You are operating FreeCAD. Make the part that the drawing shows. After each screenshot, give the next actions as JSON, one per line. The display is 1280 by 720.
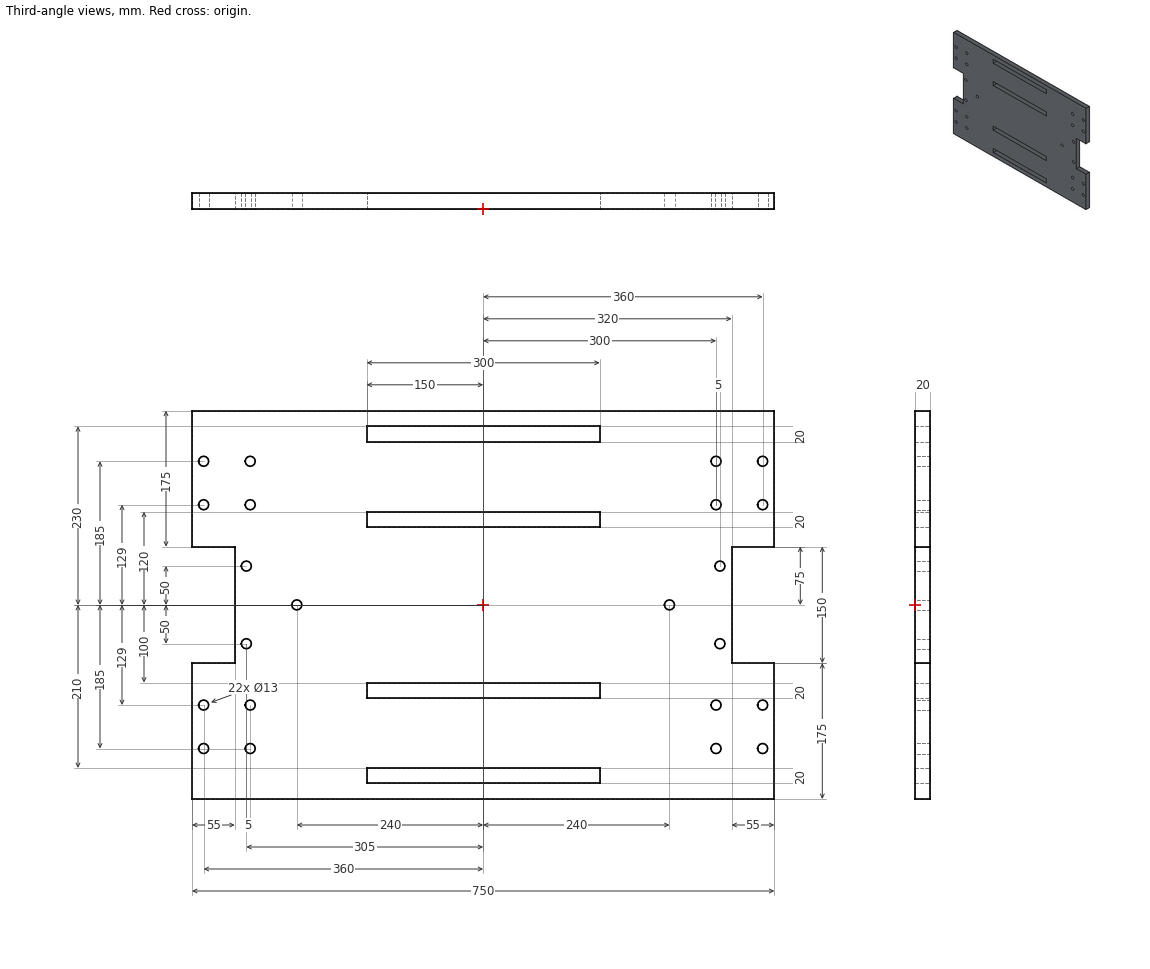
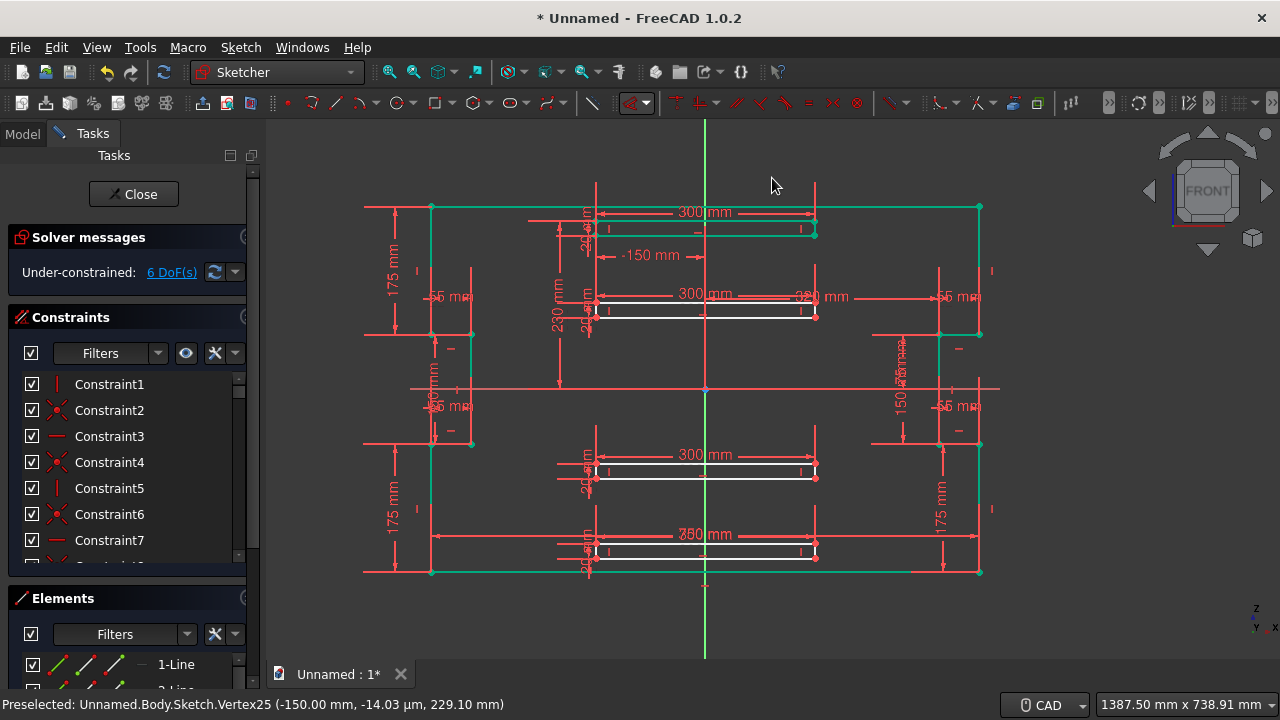
{"action": "left_click", "coordinate": [596, 303]}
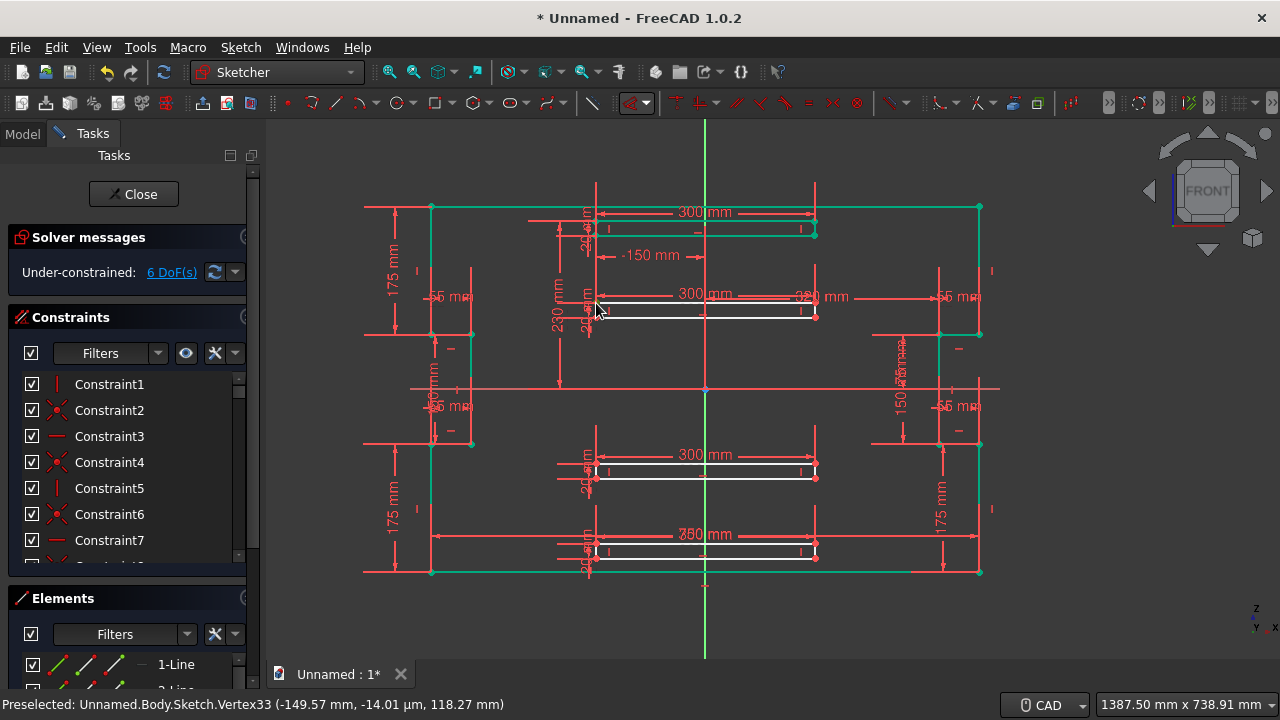
{"action": "left_click", "coordinate": [648, 104]}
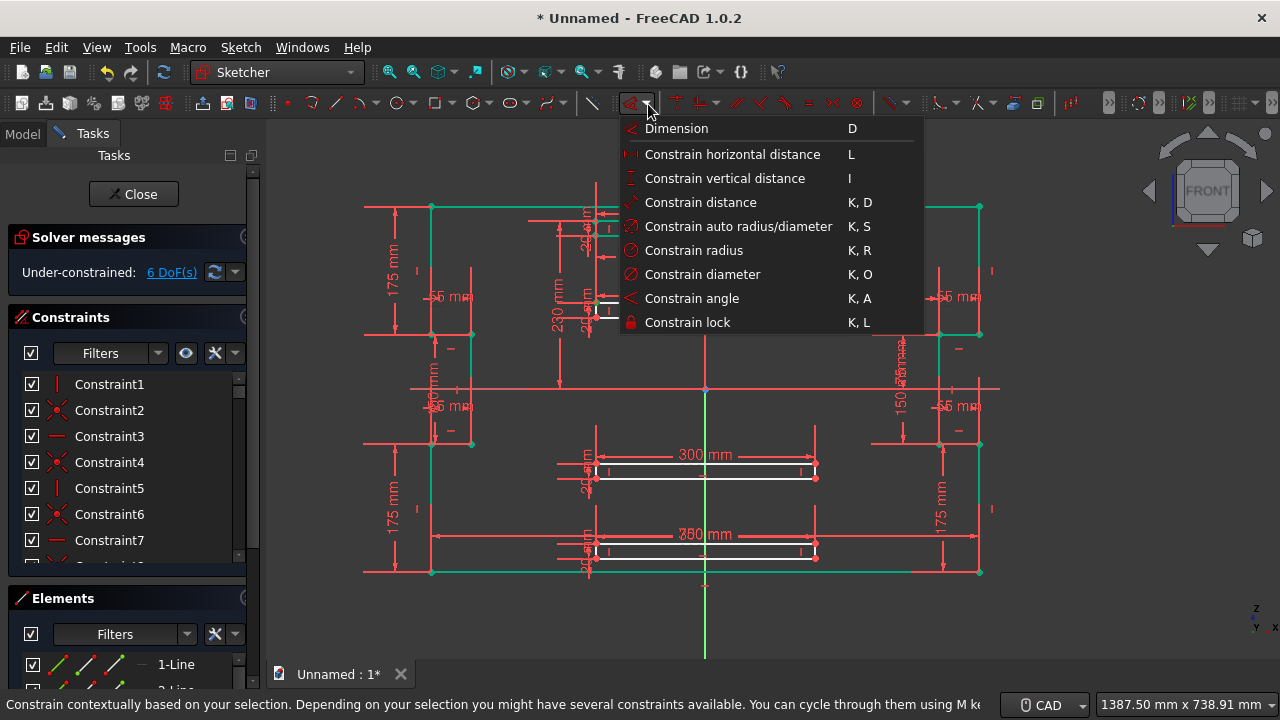
{"action": "left_click", "coordinate": [772, 154]}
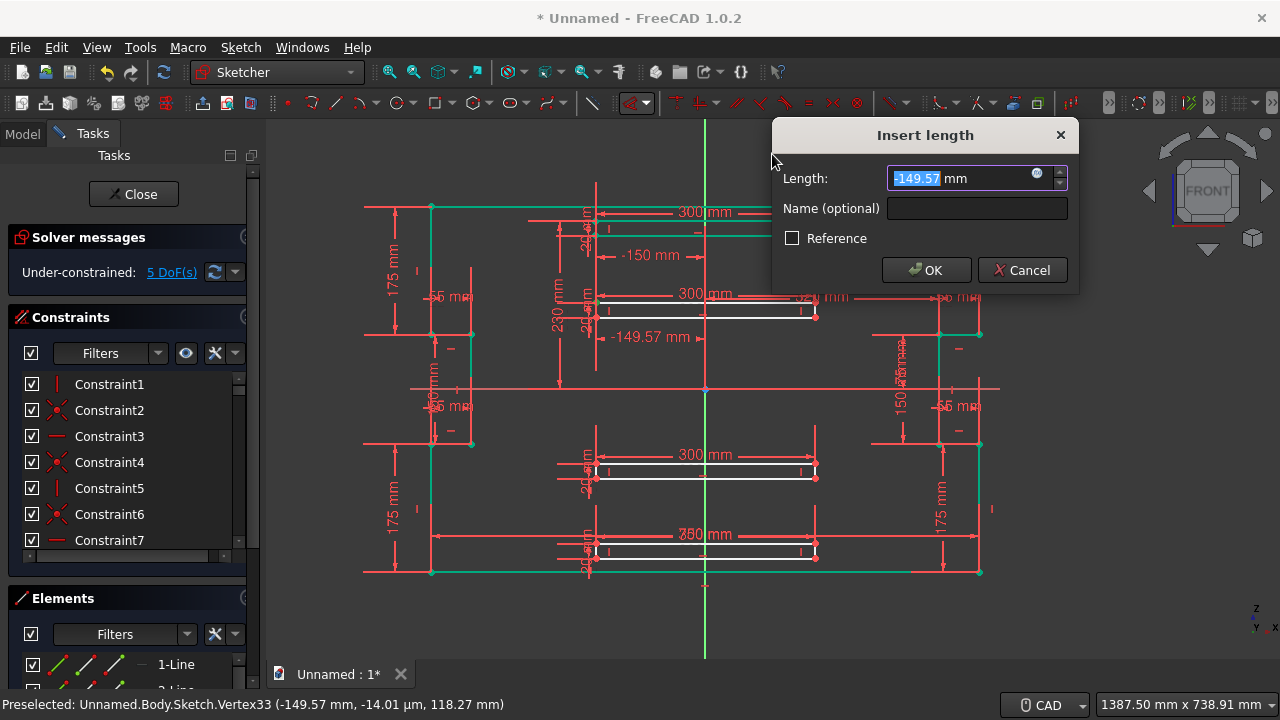
{"action": "type", "text": "-150"}
{"action": "key", "text": "Return"}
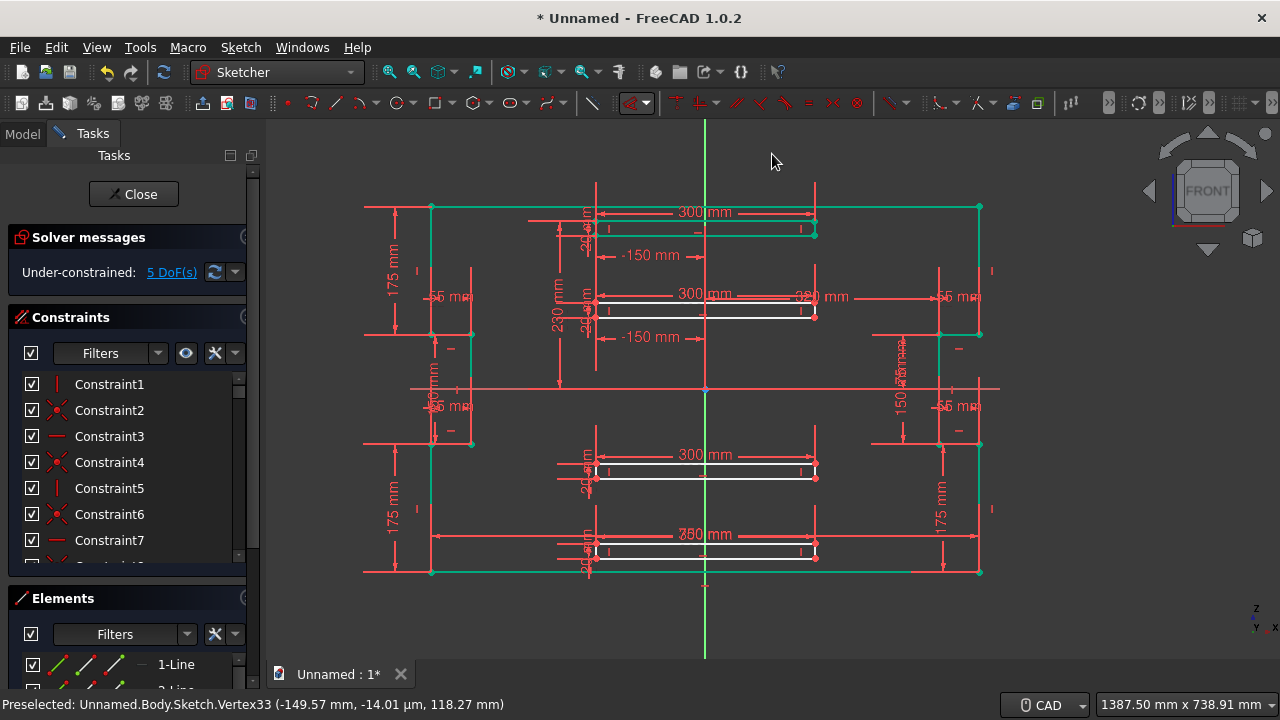
{"action": "left_click", "coordinate": [596, 303]}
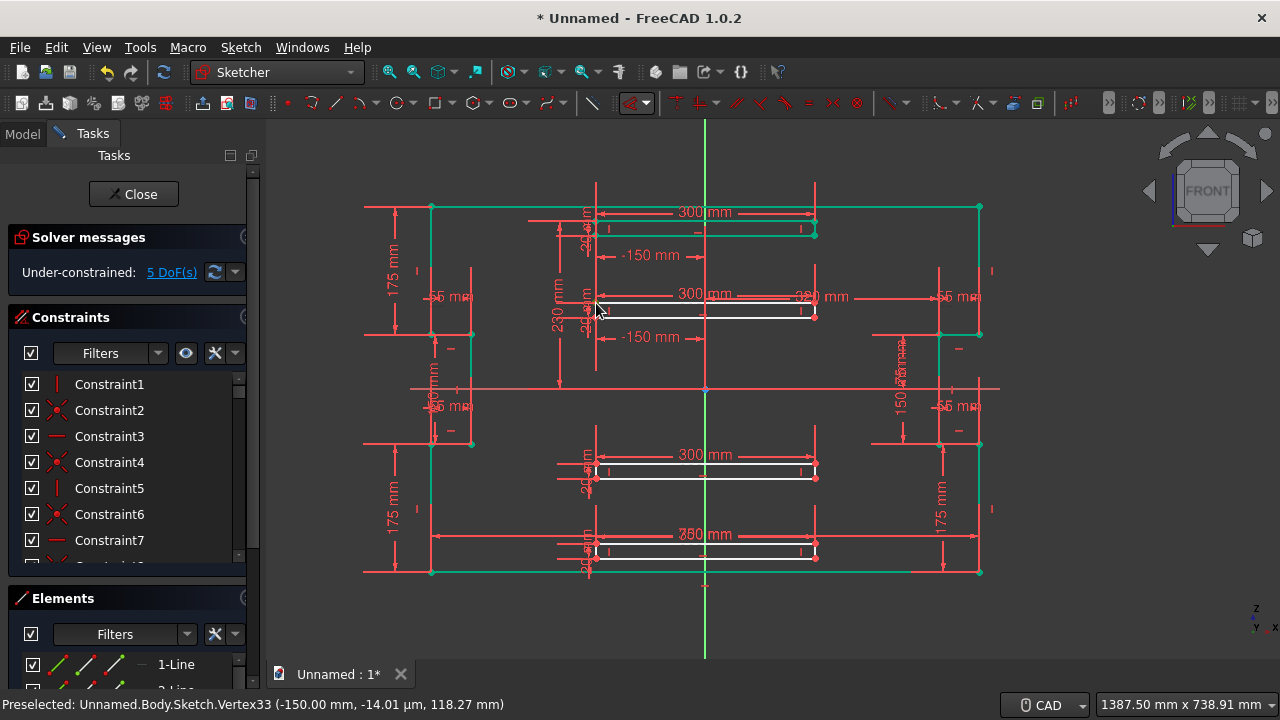
{"action": "key", "text": "i"}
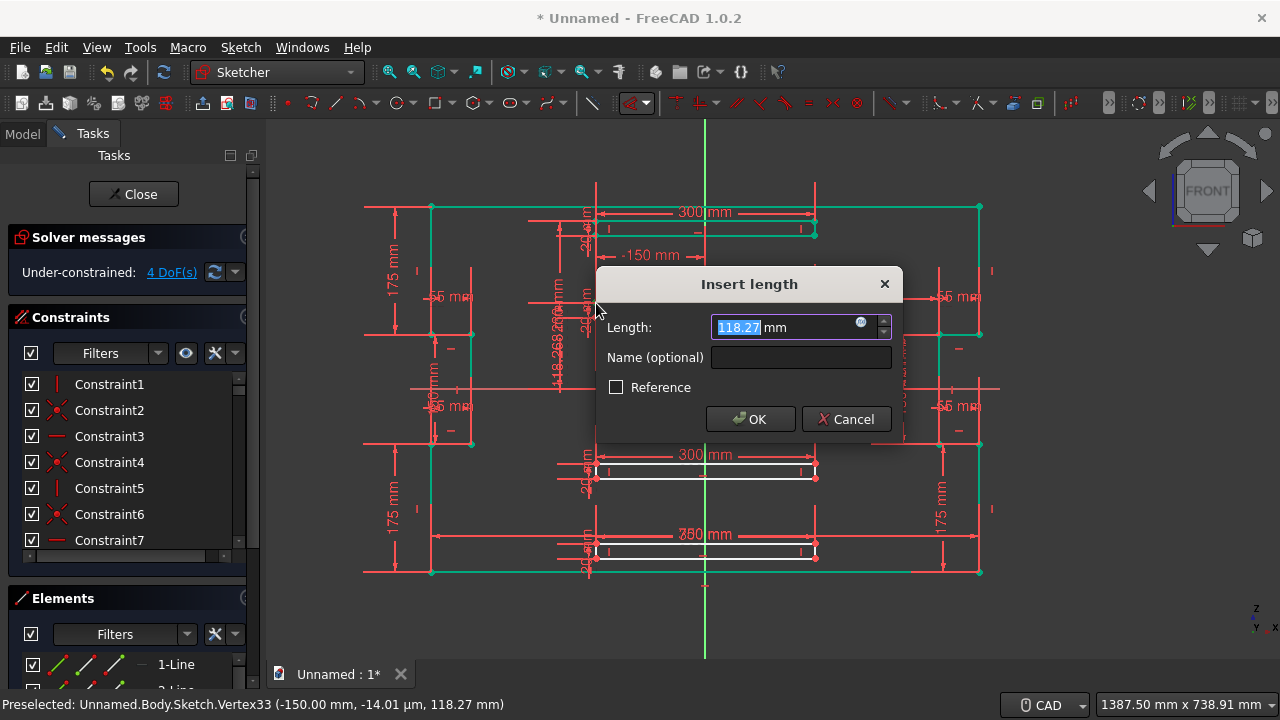
{"action": "type", "text": "120"}
{"action": "key", "text": "Return"}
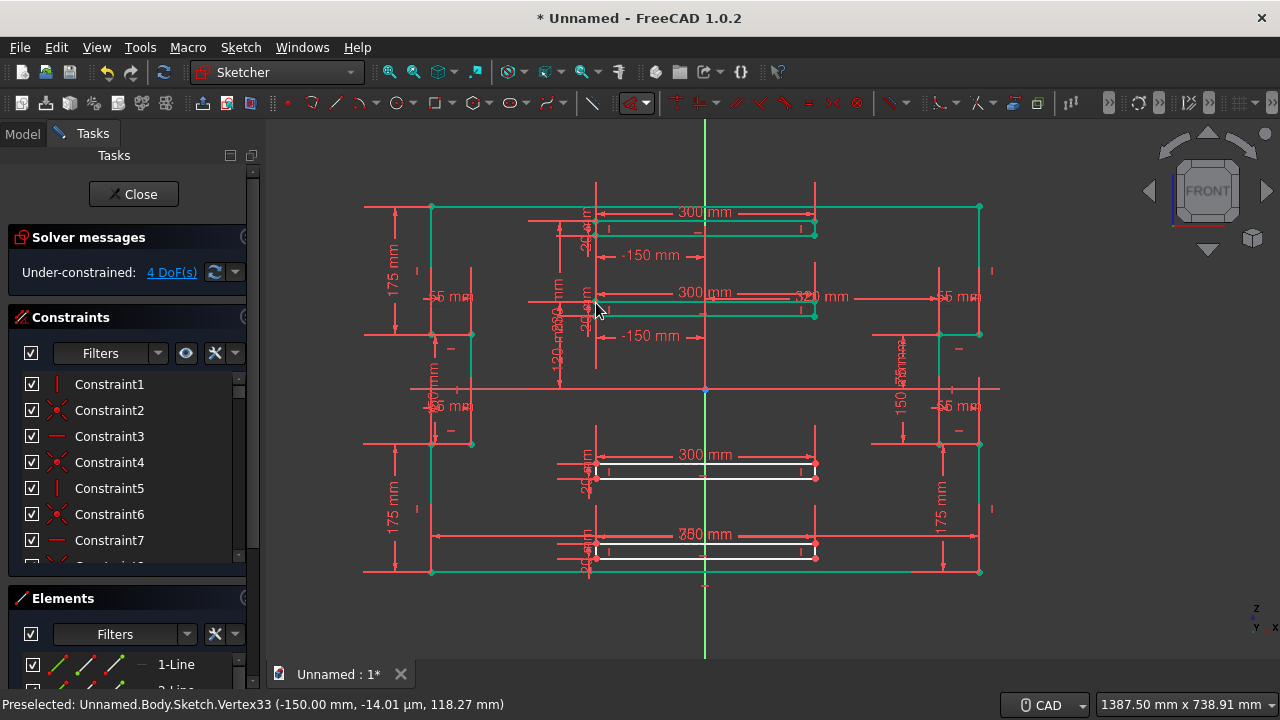
{"action": "left_click", "coordinate": [596, 464]}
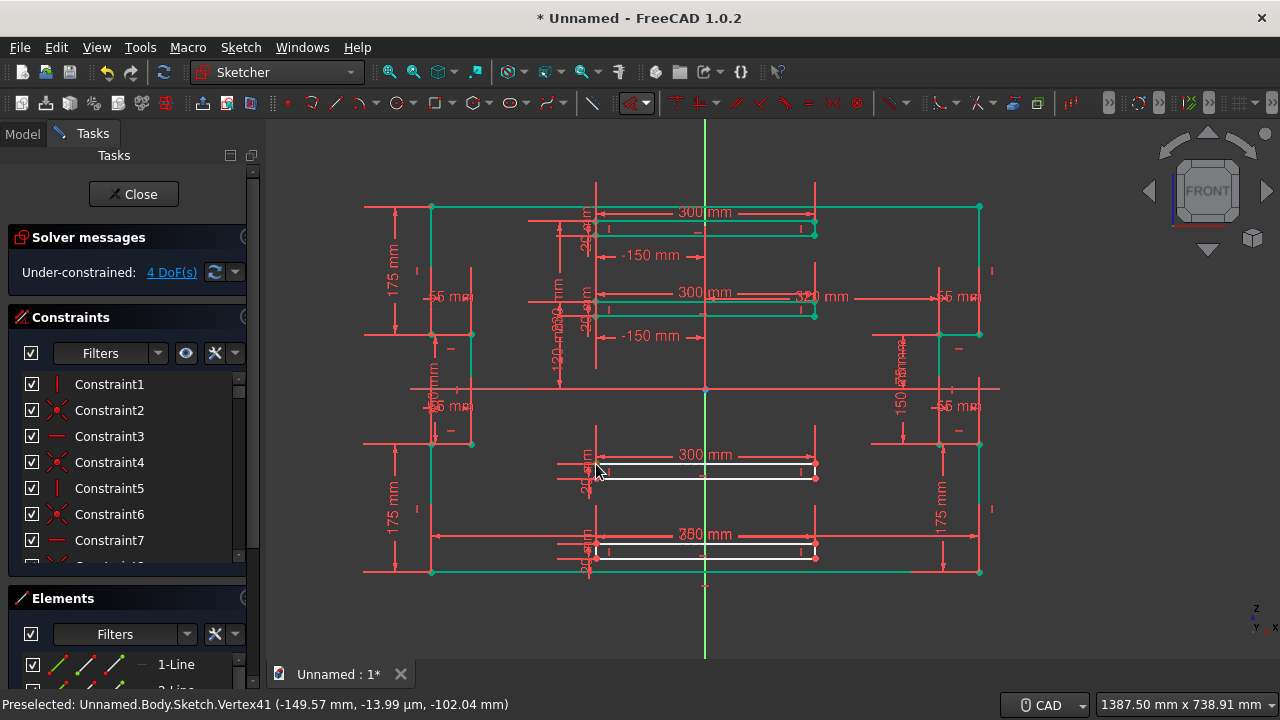
{"action": "left_click", "coordinate": [648, 104]}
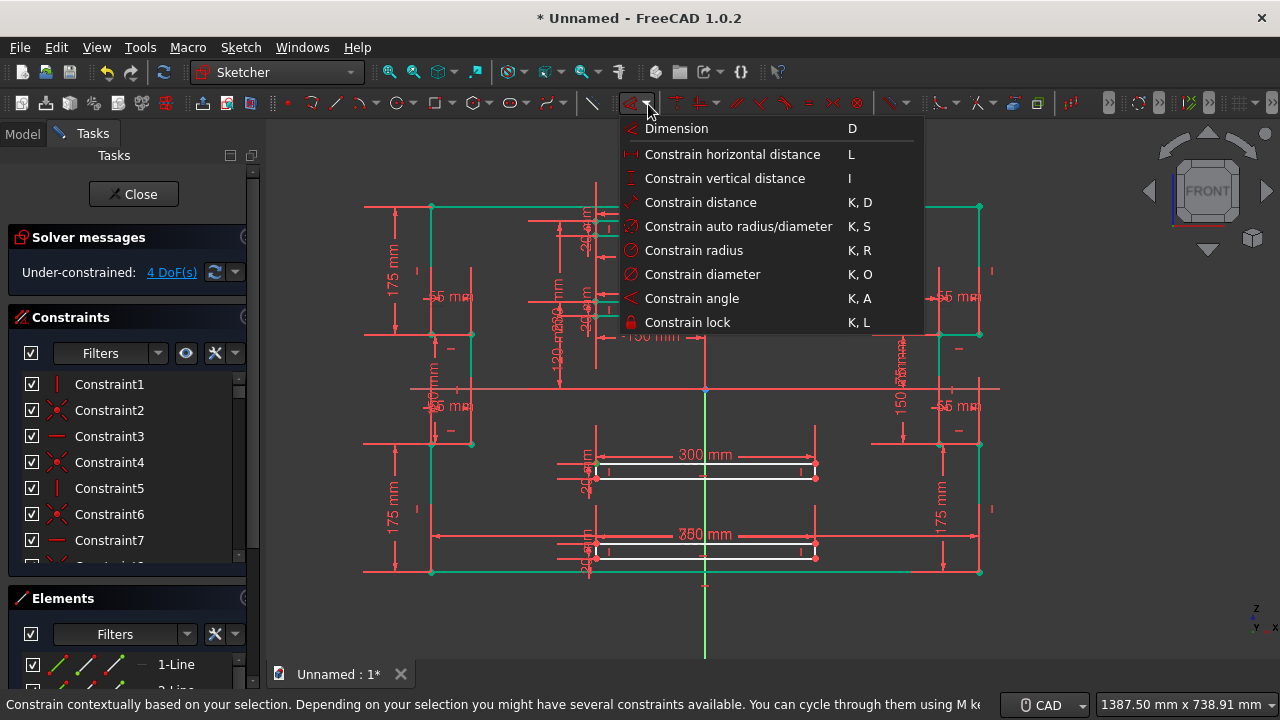
{"action": "left_click", "coordinate": [772, 154]}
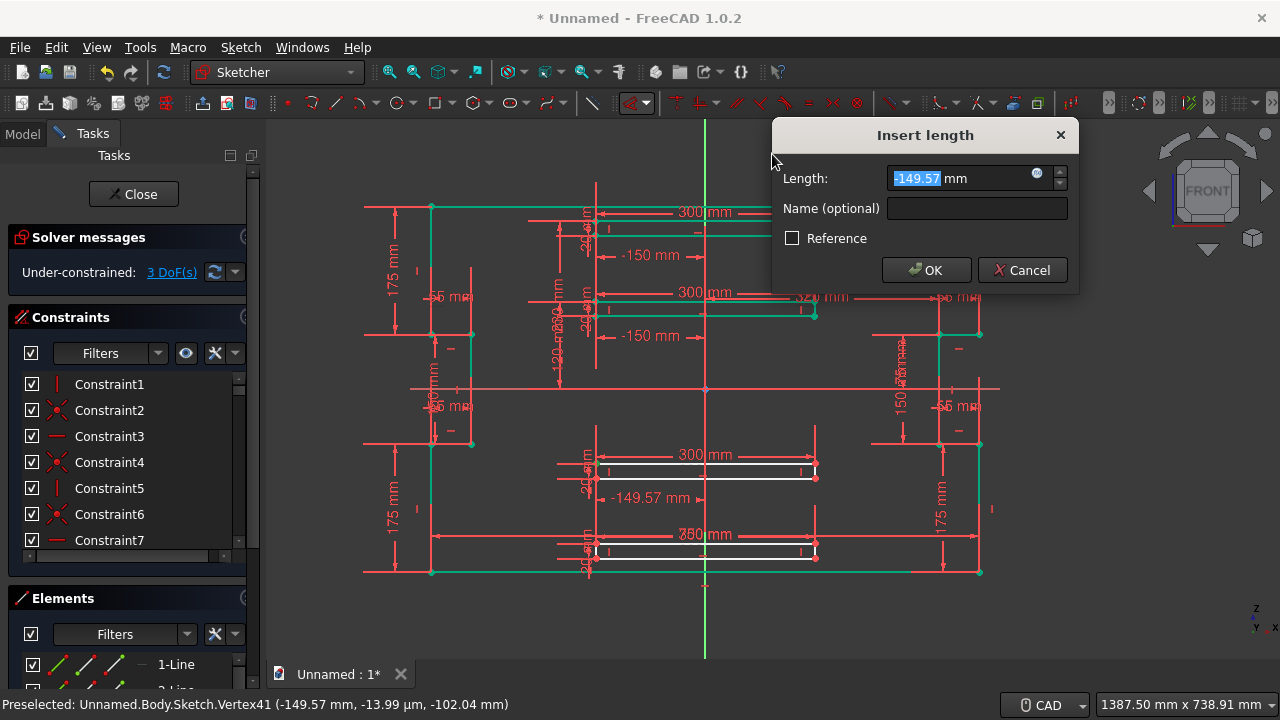
{"action": "type", "text": "-150"}
{"action": "key", "text": "Return"}